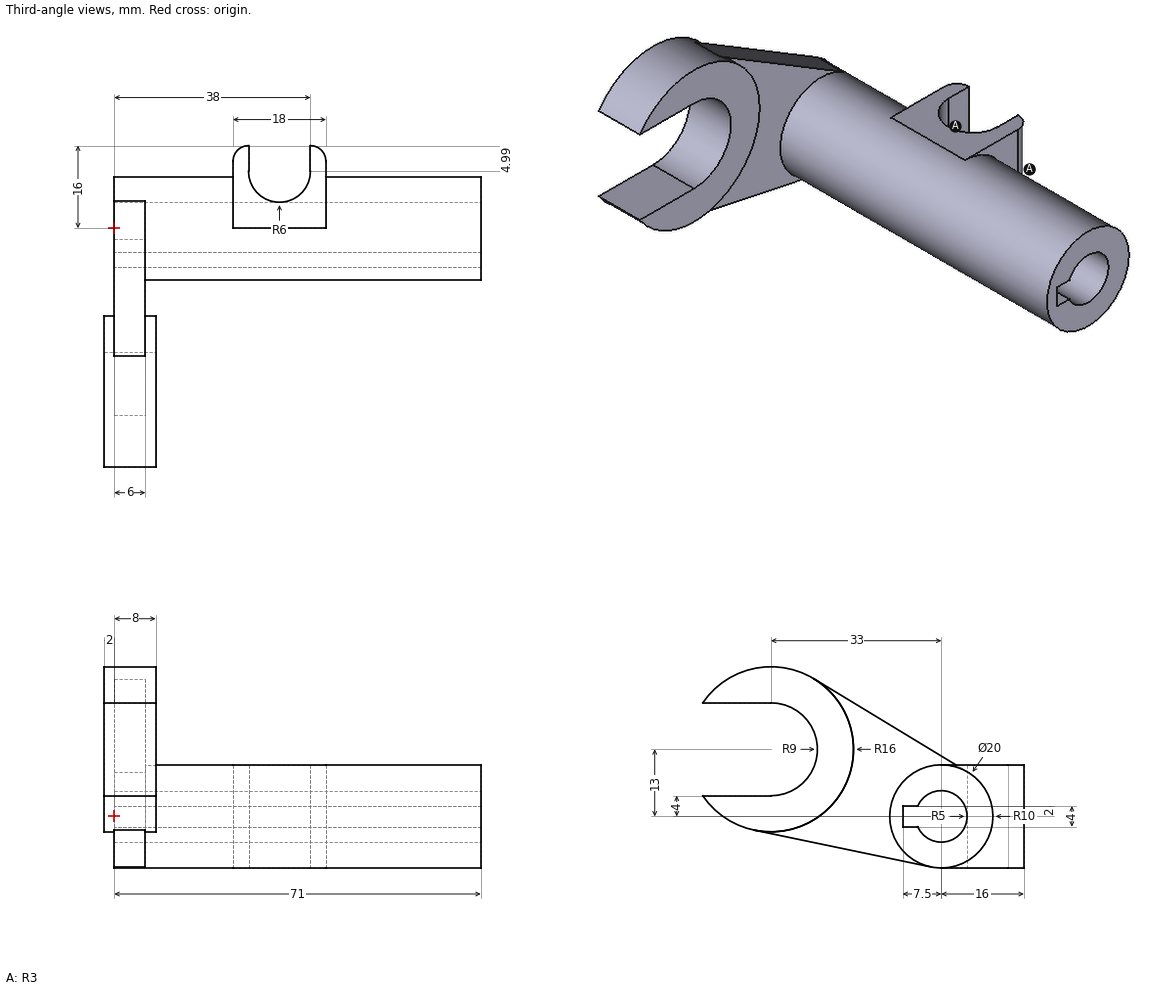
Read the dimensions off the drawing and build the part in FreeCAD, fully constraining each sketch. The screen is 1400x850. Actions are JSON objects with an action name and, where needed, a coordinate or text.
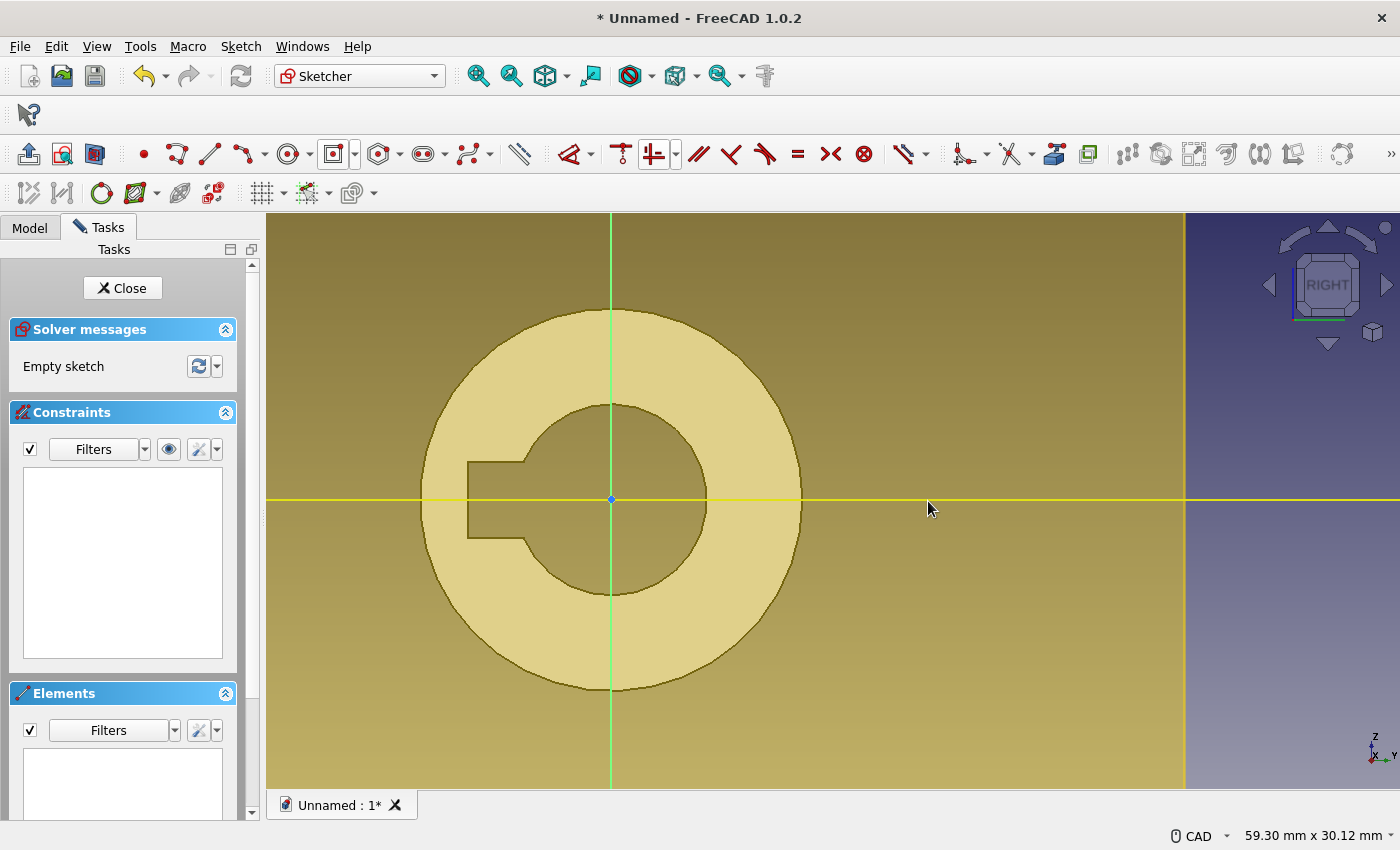
{"action": "left_click", "coordinate": [177, 154]}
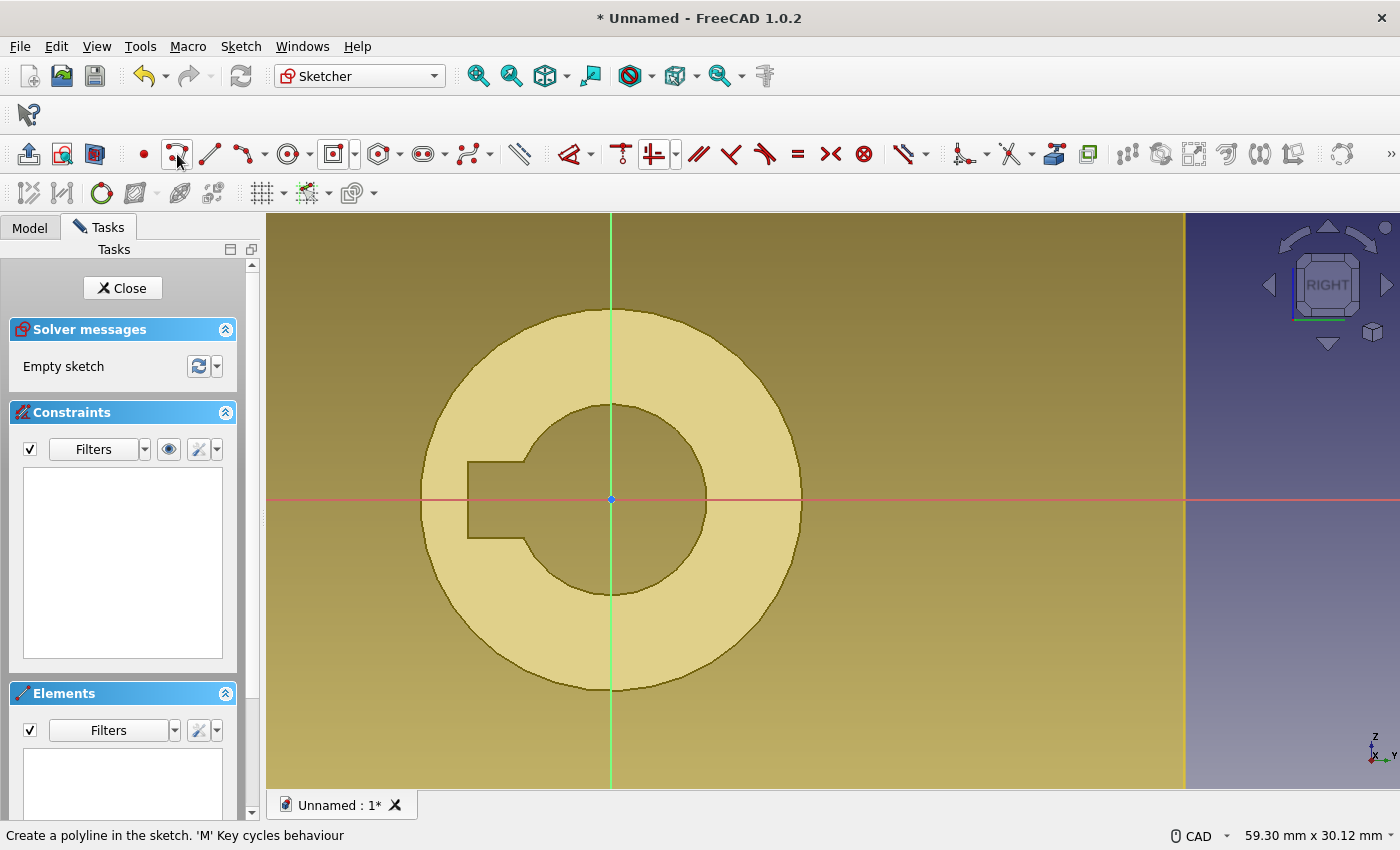
{"action": "left_click", "coordinate": [611, 691]}
{"action": "left_click", "coordinate": [917, 691]}
{"action": "left_click", "coordinate": [917, 309]}
{"action": "left_click", "coordinate": [611, 309]}
{"action": "right_click", "coordinate": [611, 309]}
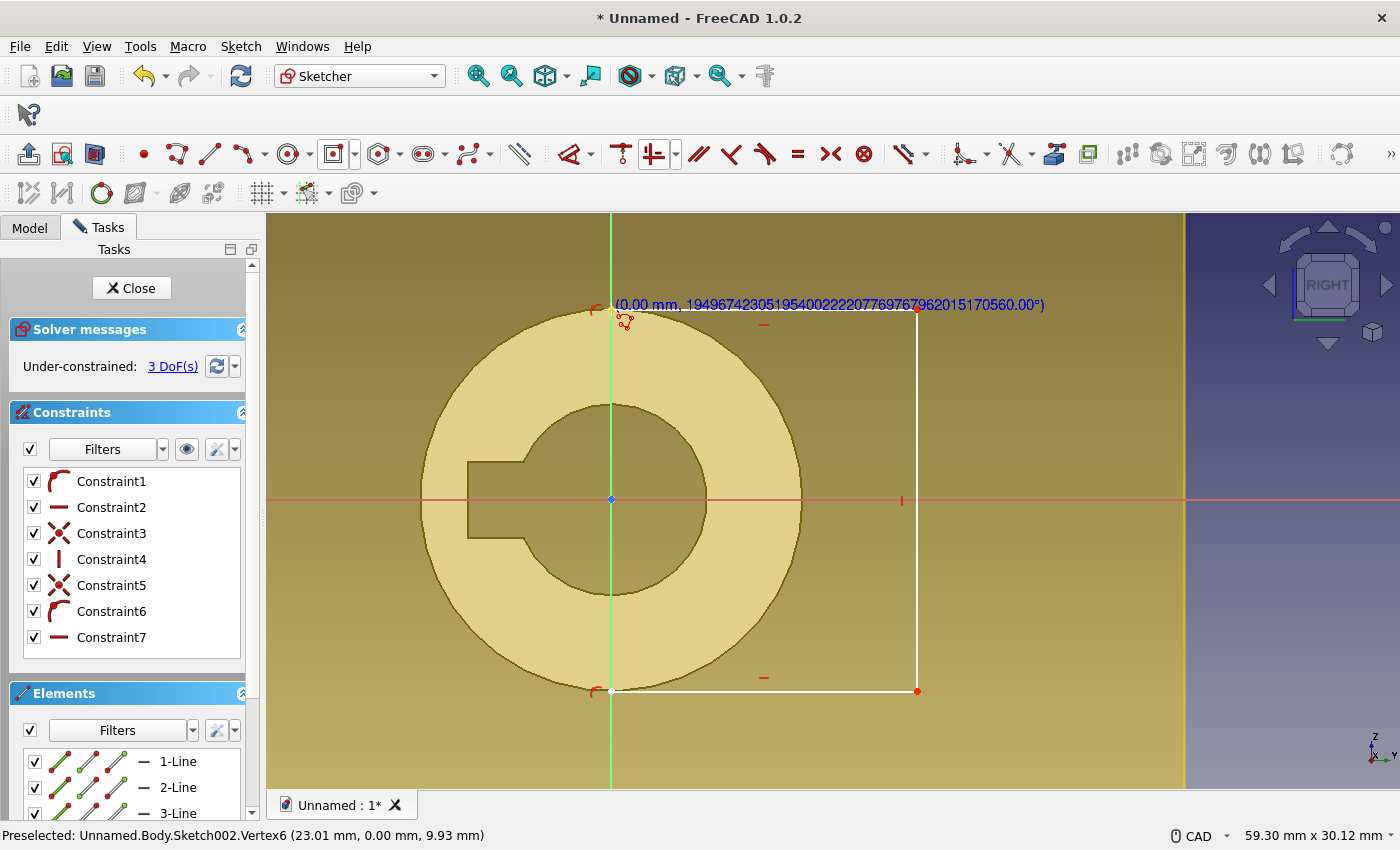
{"action": "key", "text": "g 3 a"}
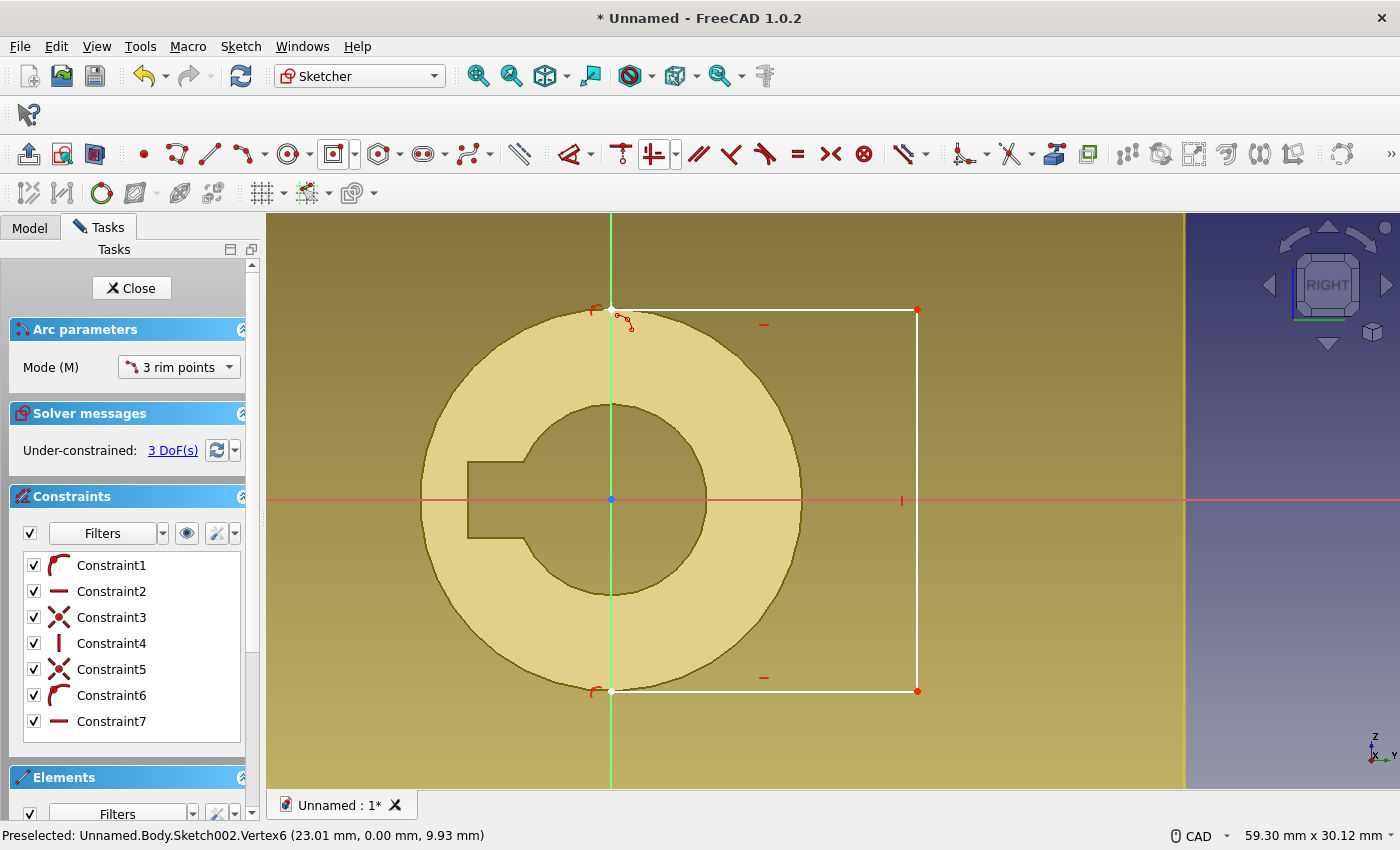
{"action": "left_click", "coordinate": [611, 310]}
{"action": "left_click", "coordinate": [611, 692]}
{"action": "left_click", "coordinate": [793, 559]}
{"action": "key", "text": "Escape"}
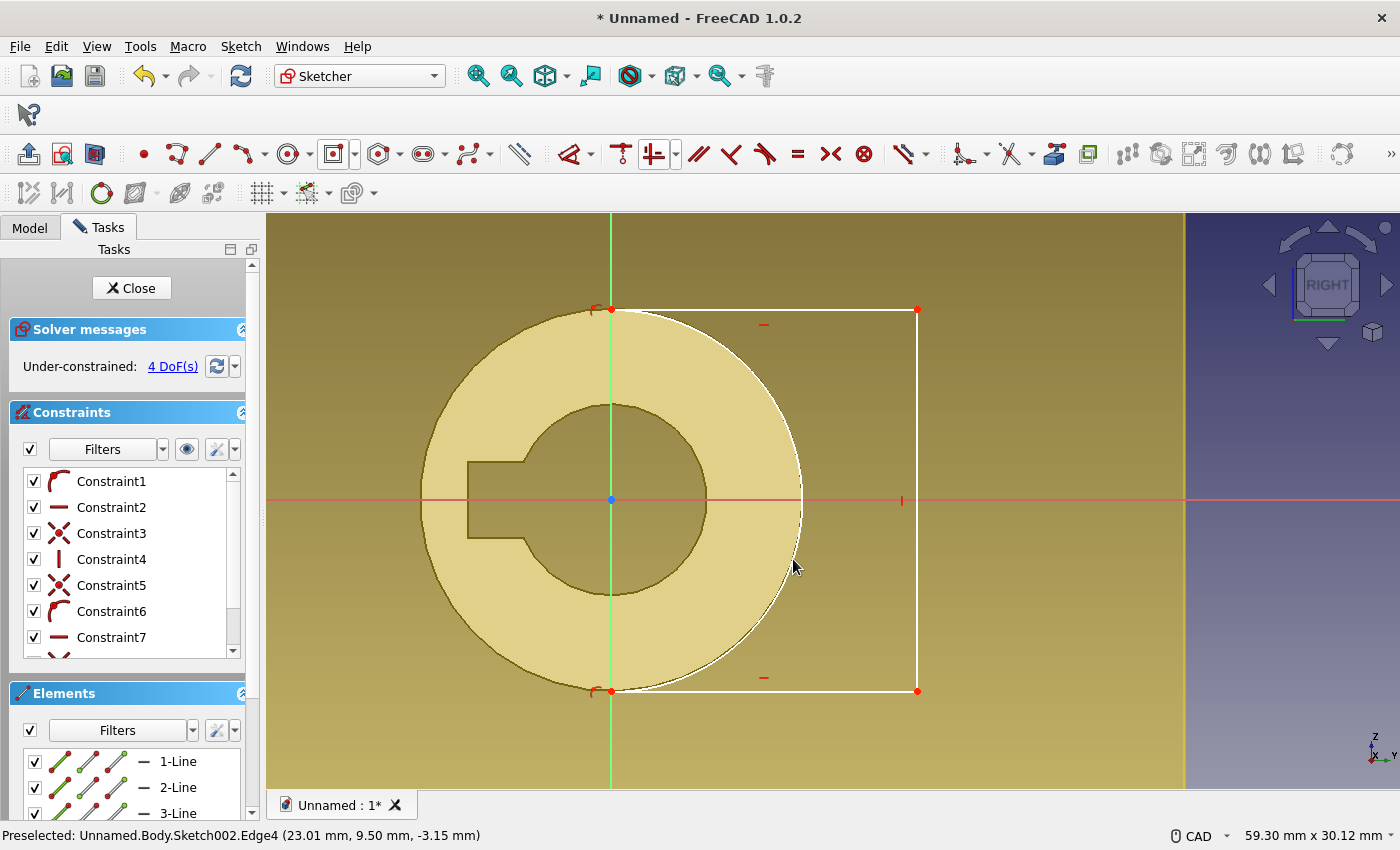
{"action": "left_click", "coordinate": [703, 692]}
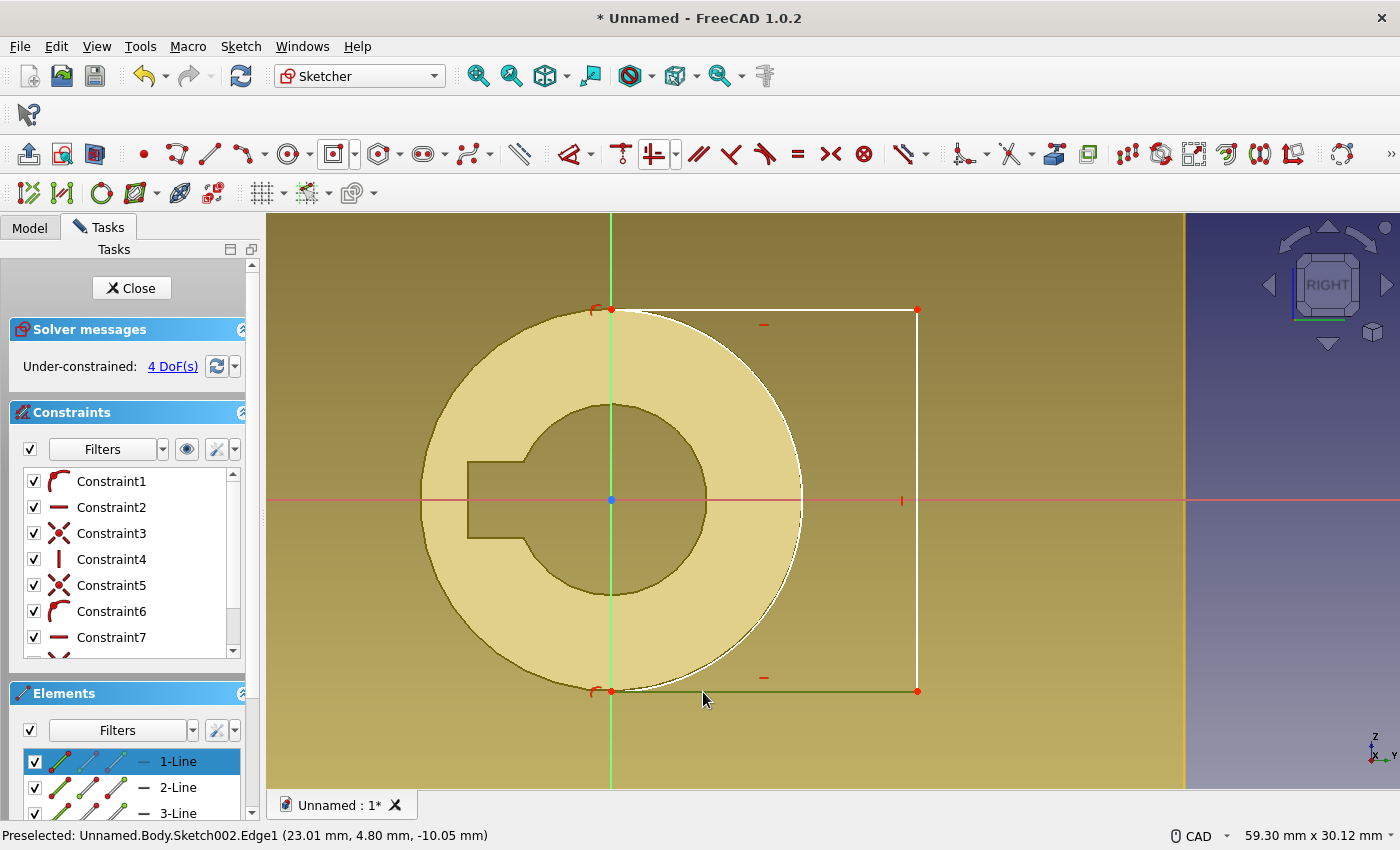
{"action": "left_click", "coordinate": [766, 613]}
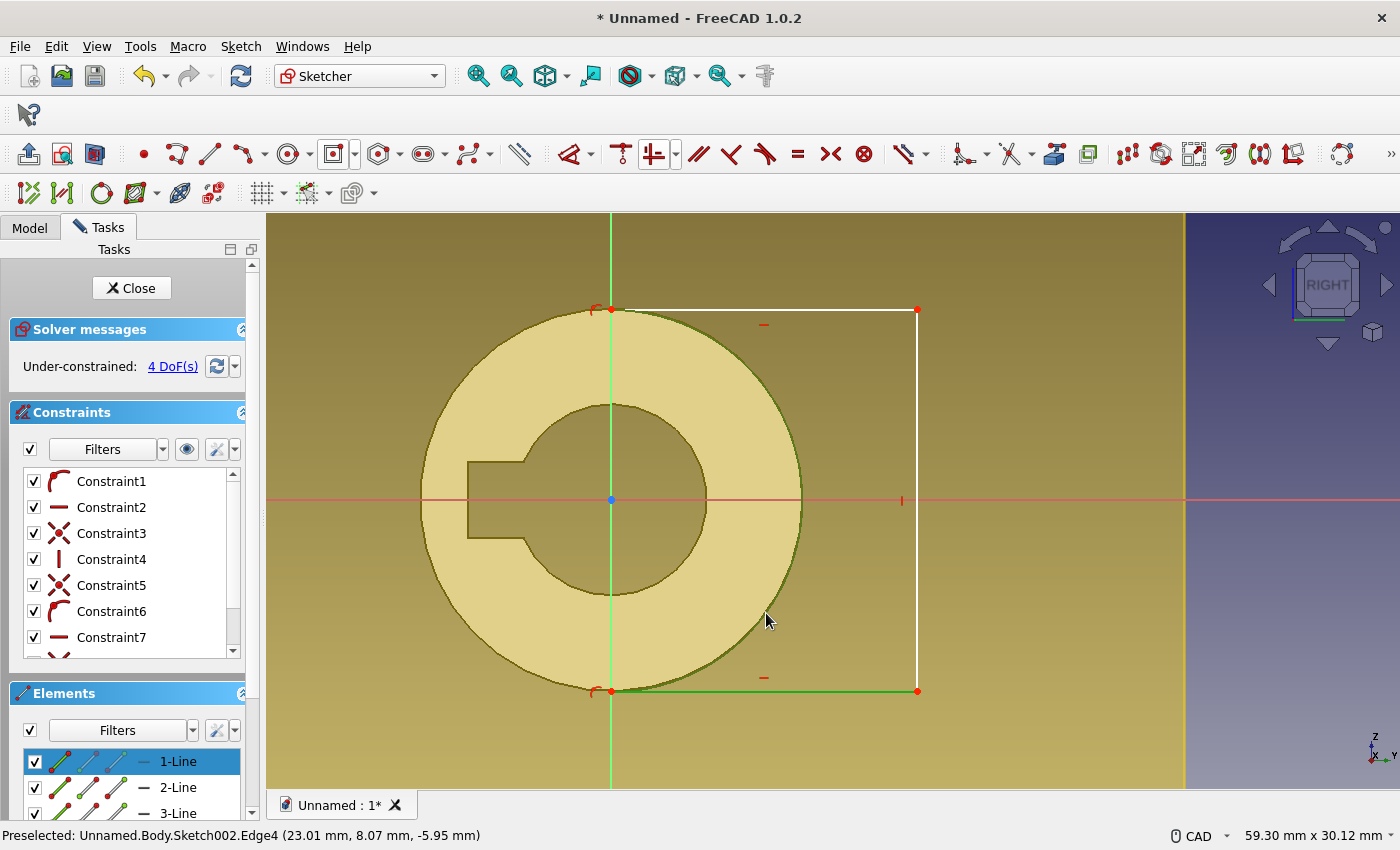
{"action": "key", "text": "t"}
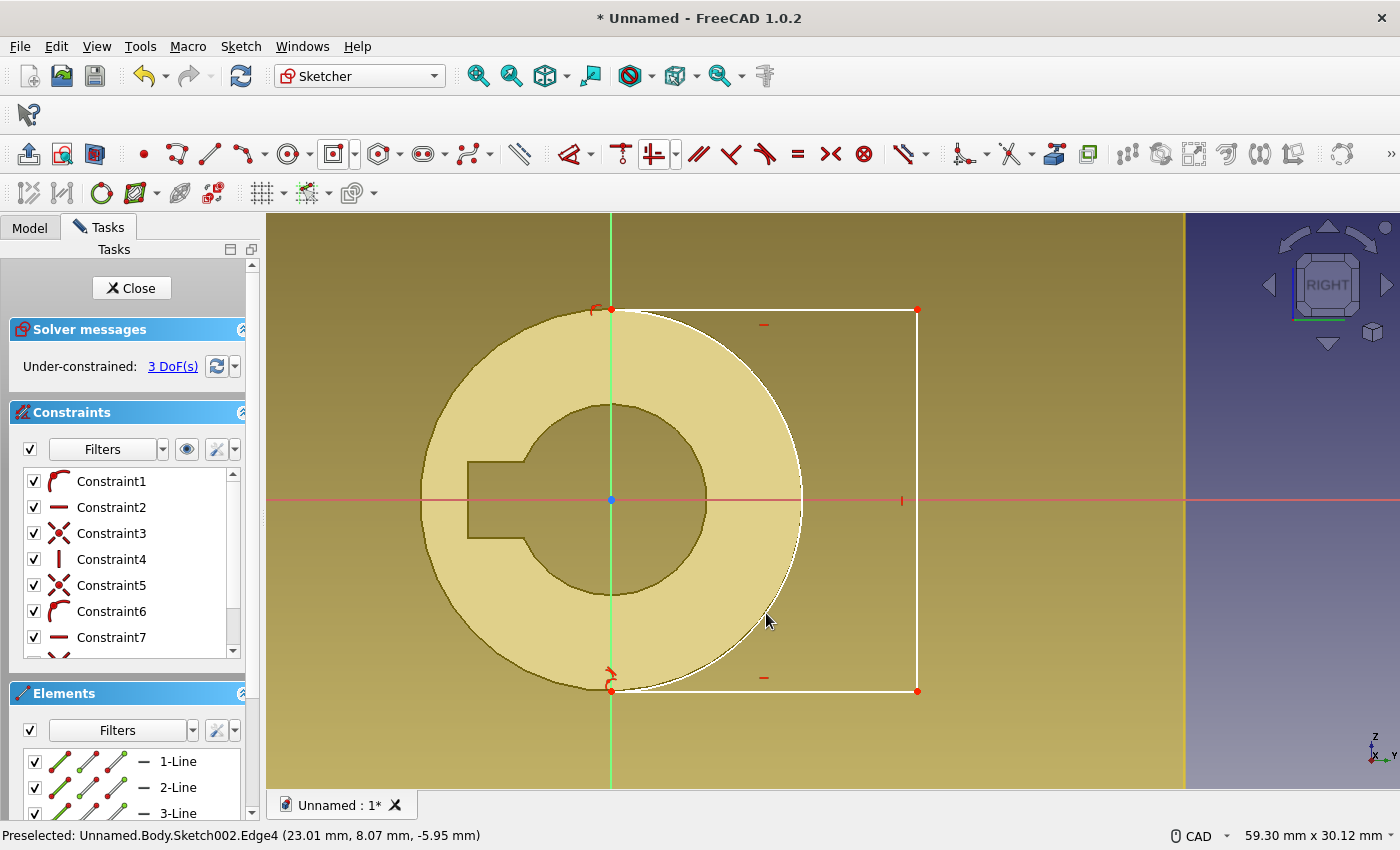
{"action": "left_click", "coordinate": [611, 501]}